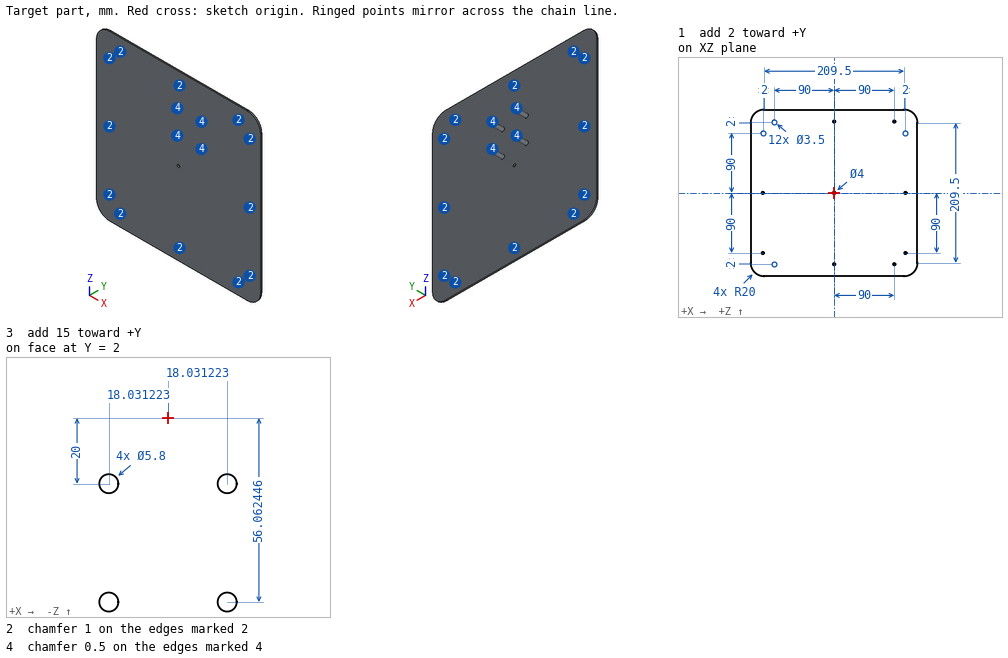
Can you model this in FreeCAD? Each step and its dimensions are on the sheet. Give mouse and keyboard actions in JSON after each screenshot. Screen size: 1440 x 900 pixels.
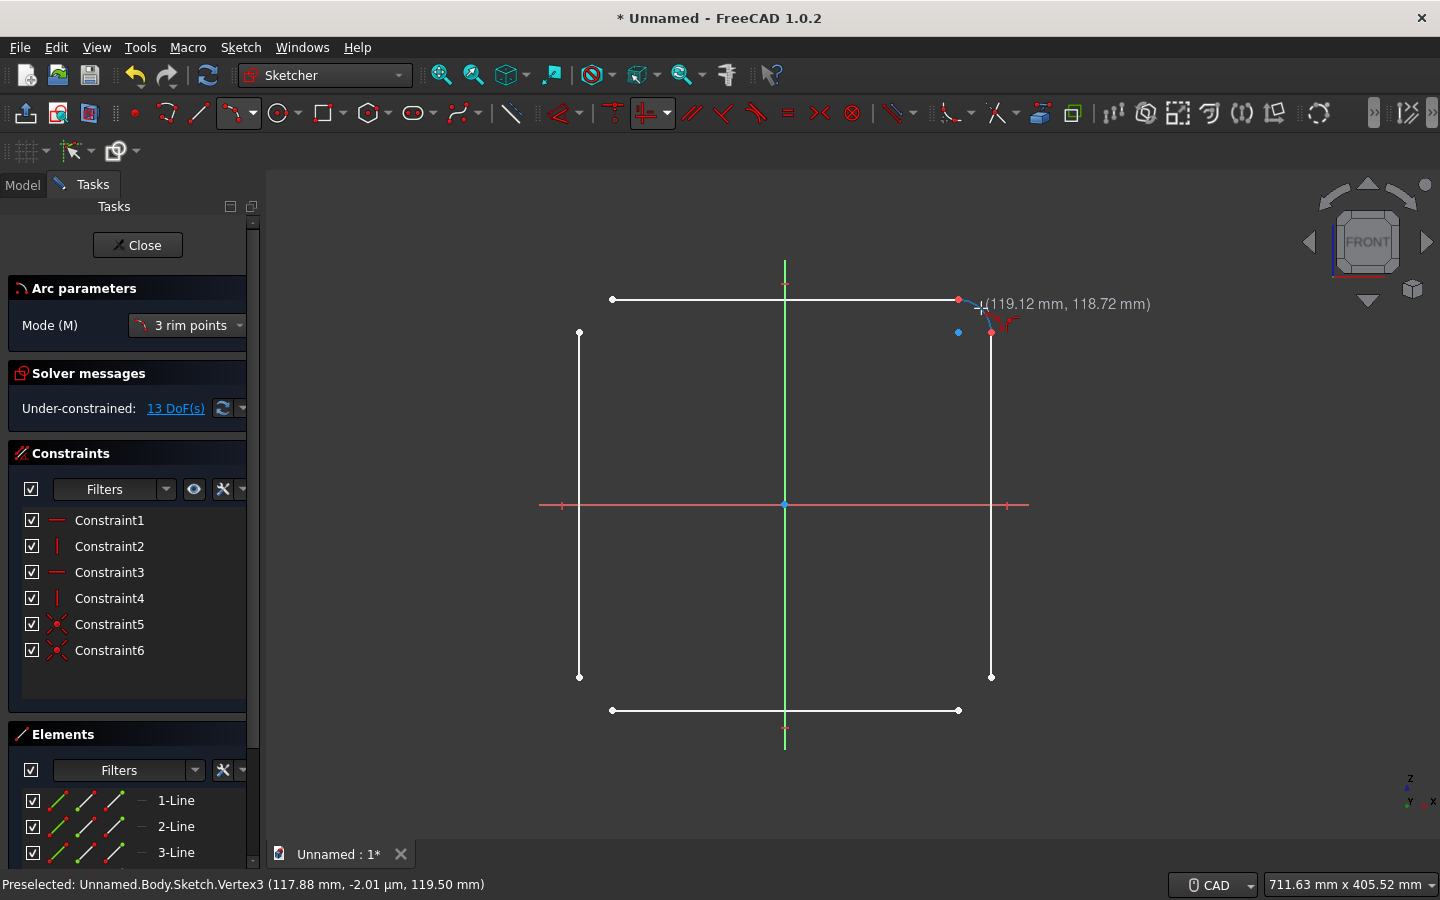
{"action": "left_click", "coordinate": [991, 678]}
{"action": "left_click", "coordinate": [958, 711]}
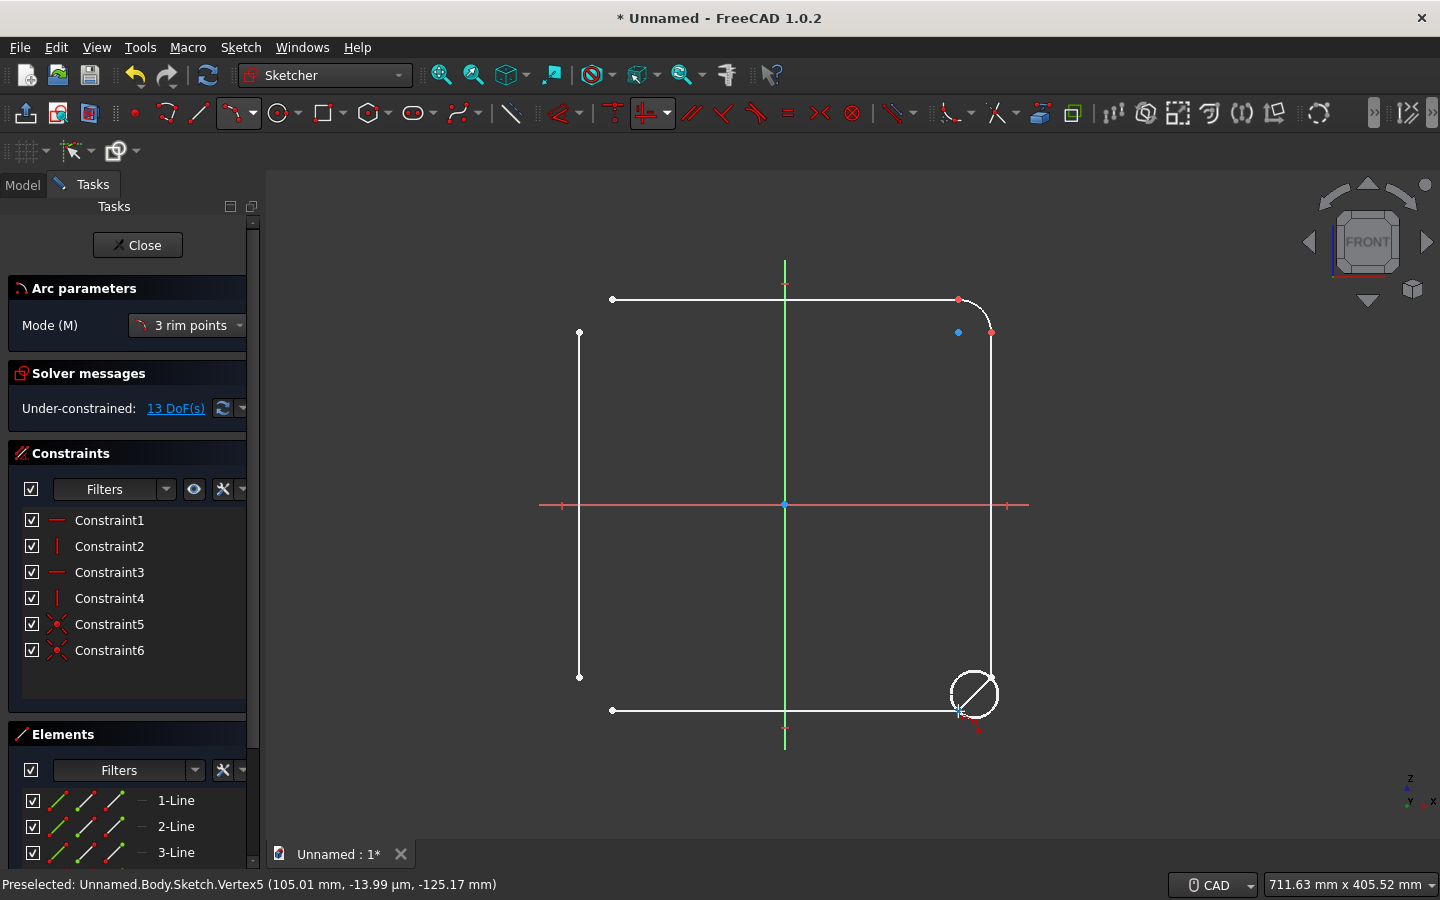
{"action": "scroll", "coordinate": [981, 701], "scroll_direction": "up", "scroll_amount": 3}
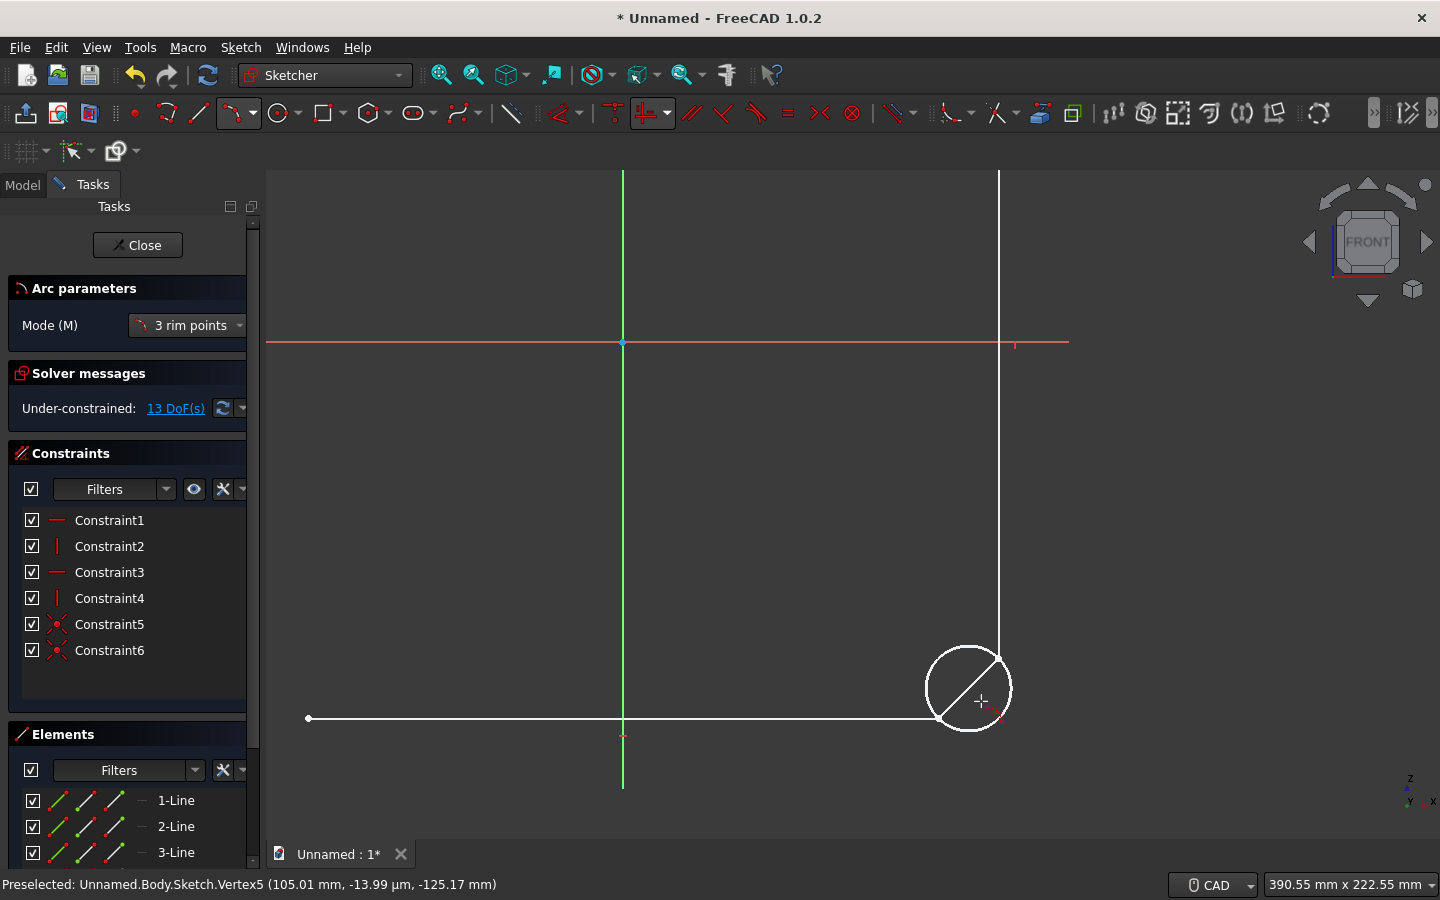
{"action": "left_click", "coordinate": [980, 700]}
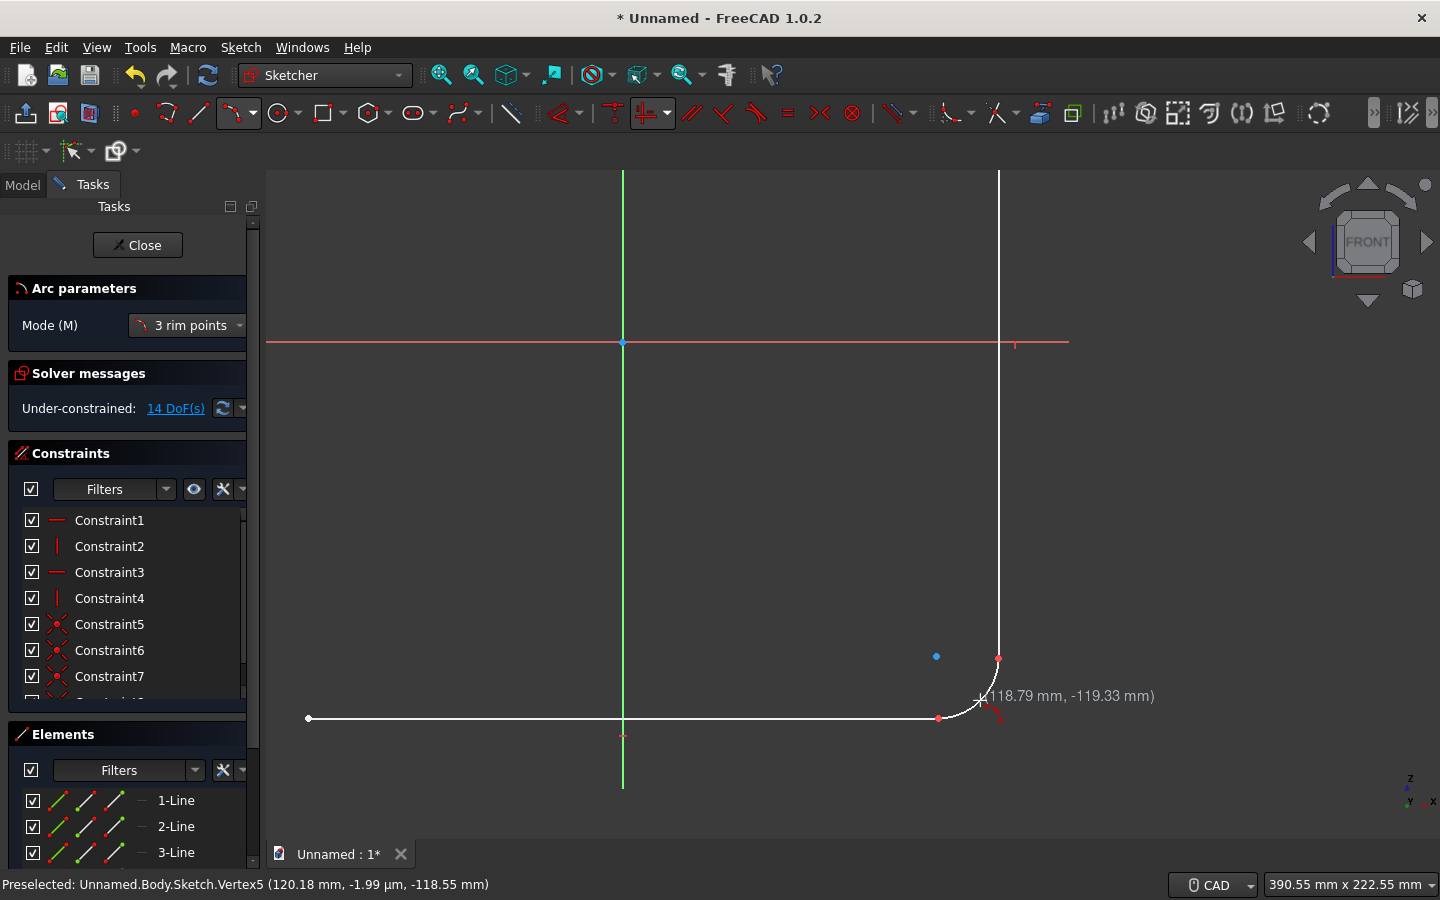
{"action": "left_click", "coordinate": [308, 719]}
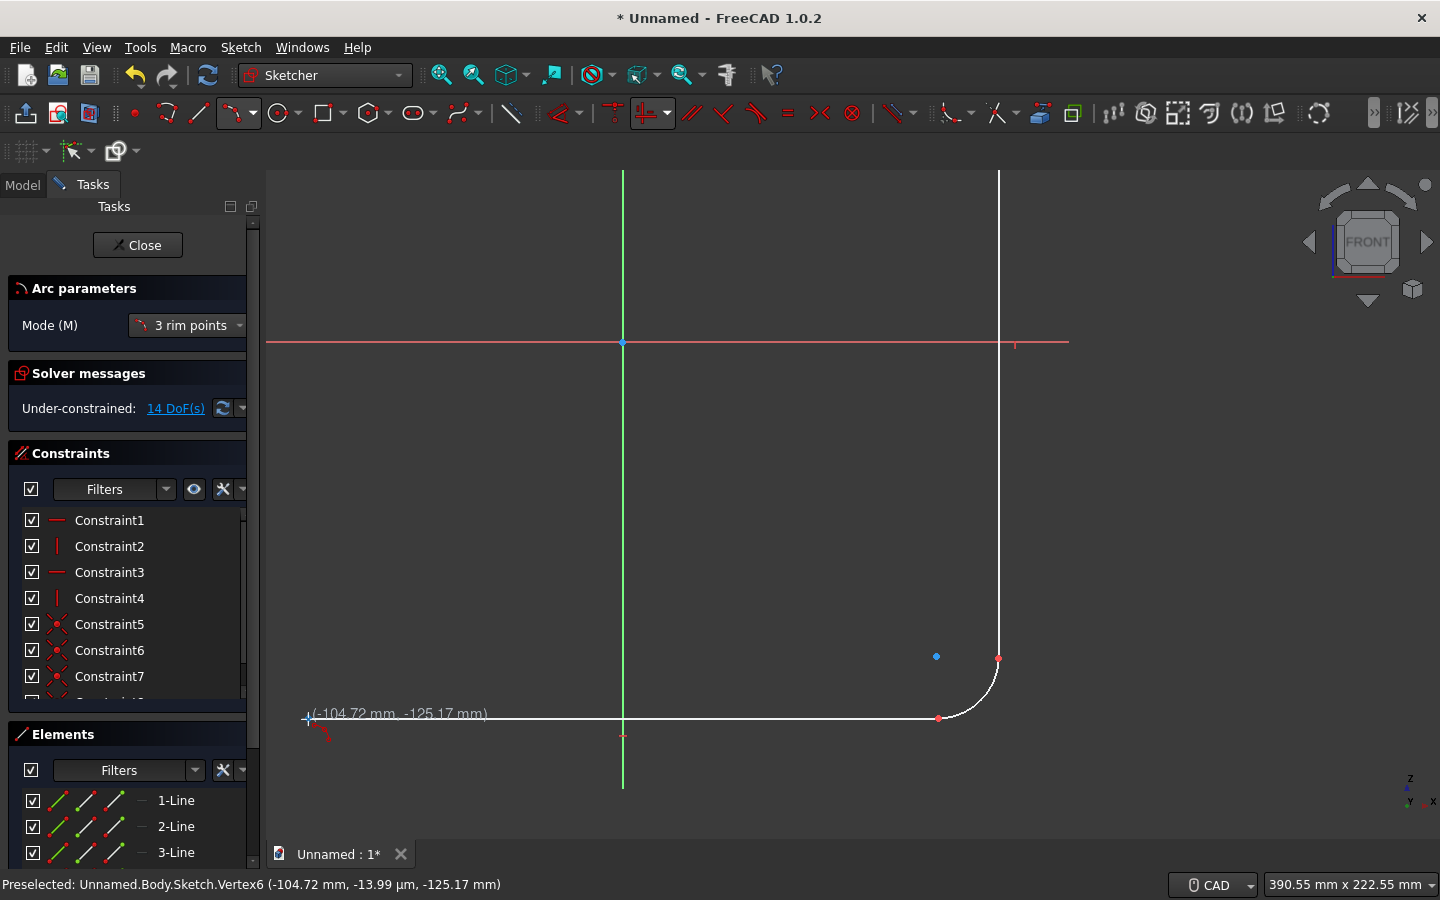
{"action": "scroll", "coordinate": [981, 702], "scroll_direction": "down", "scroll_amount": 3}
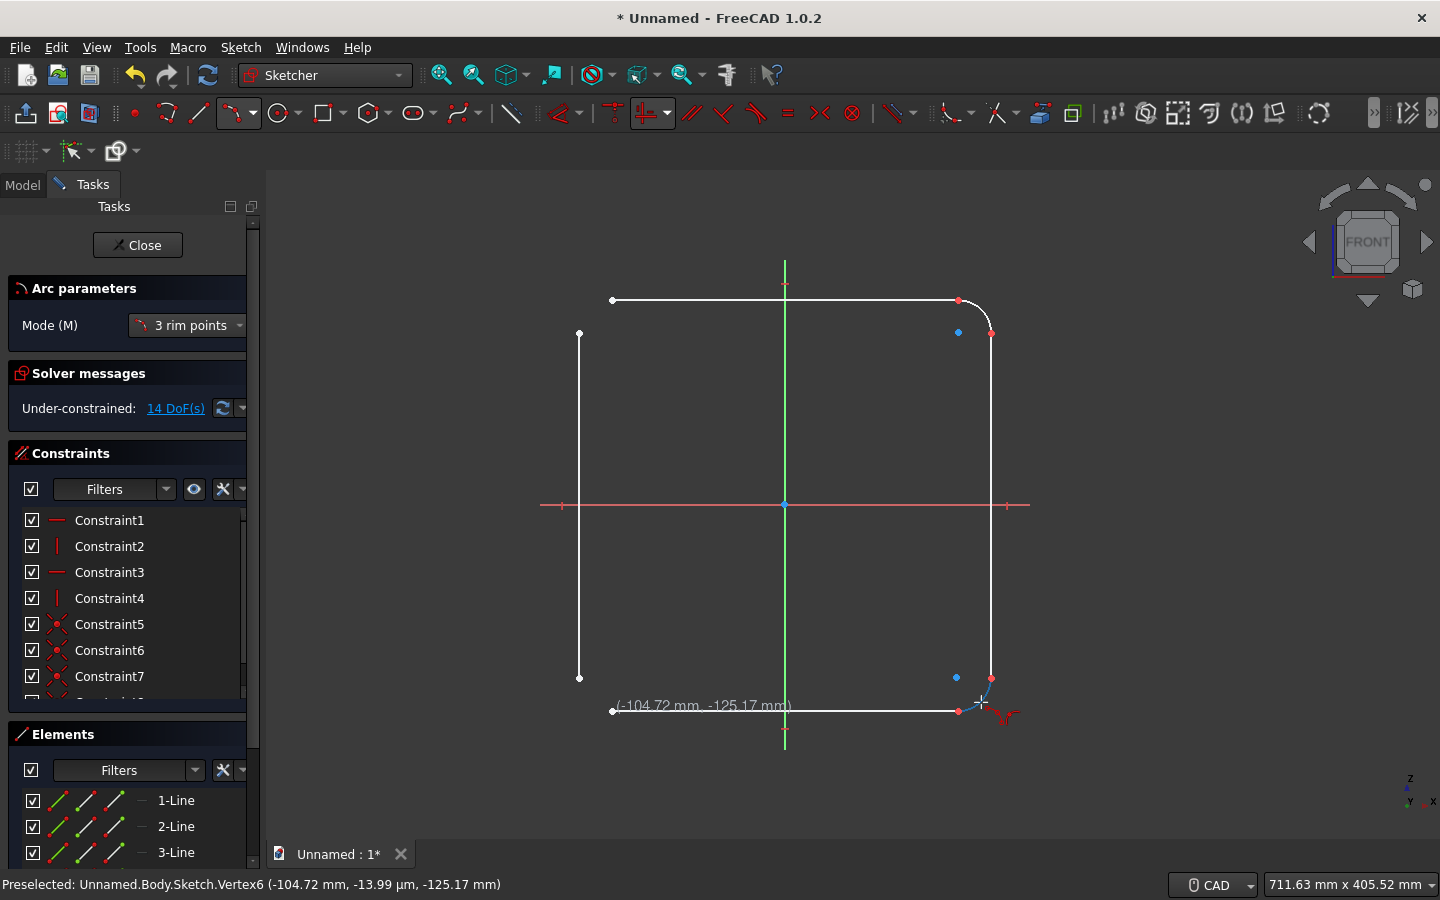
{"action": "left_click", "coordinate": [579, 678]}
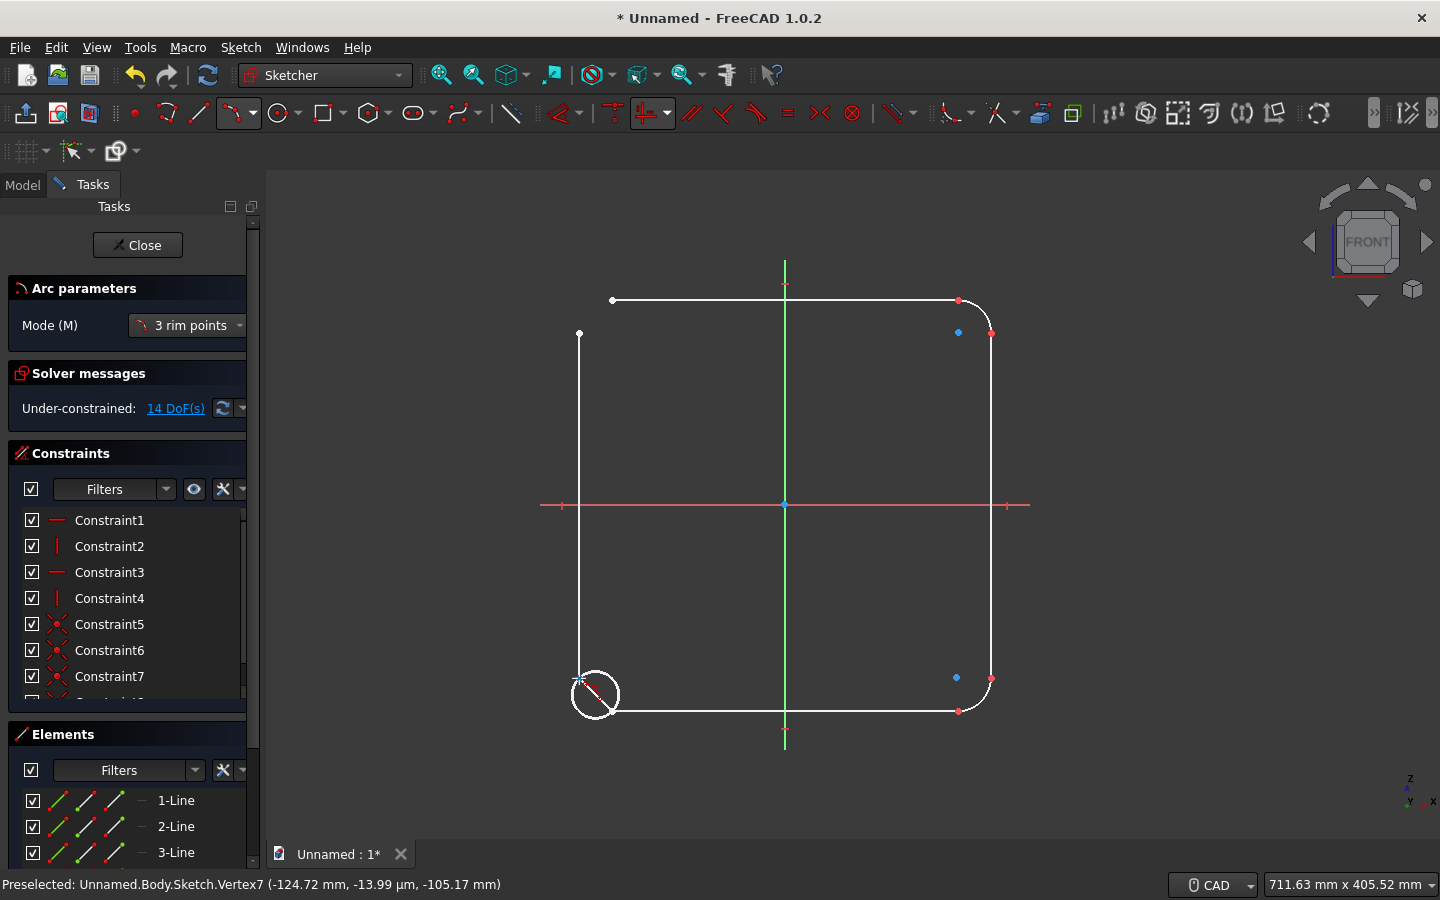
{"action": "scroll", "coordinate": [589, 701], "scroll_direction": "up", "scroll_amount": 3}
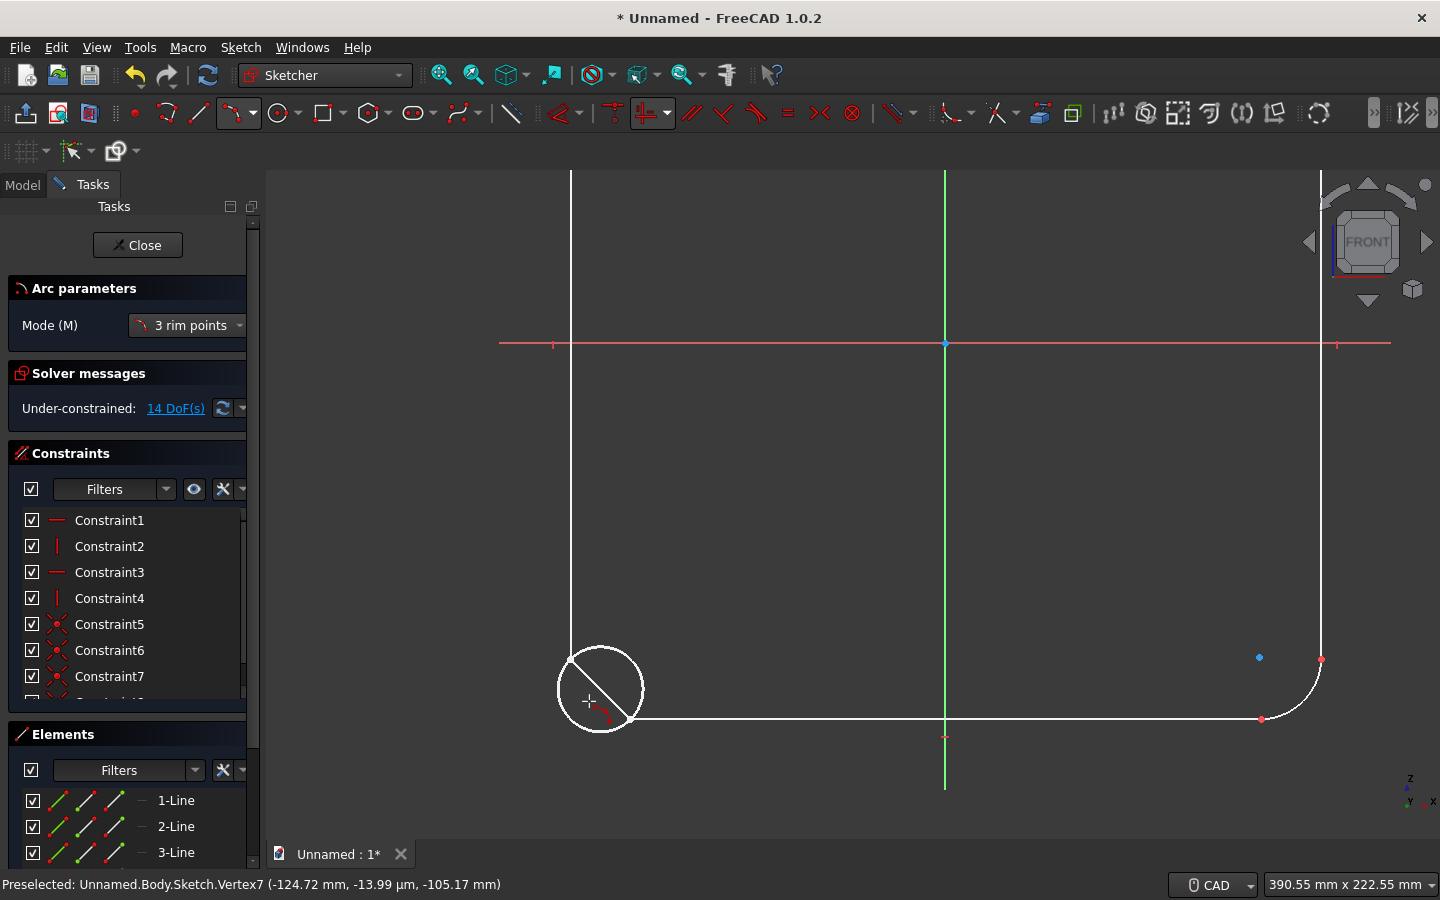
{"action": "left_click", "coordinate": [588, 701]}